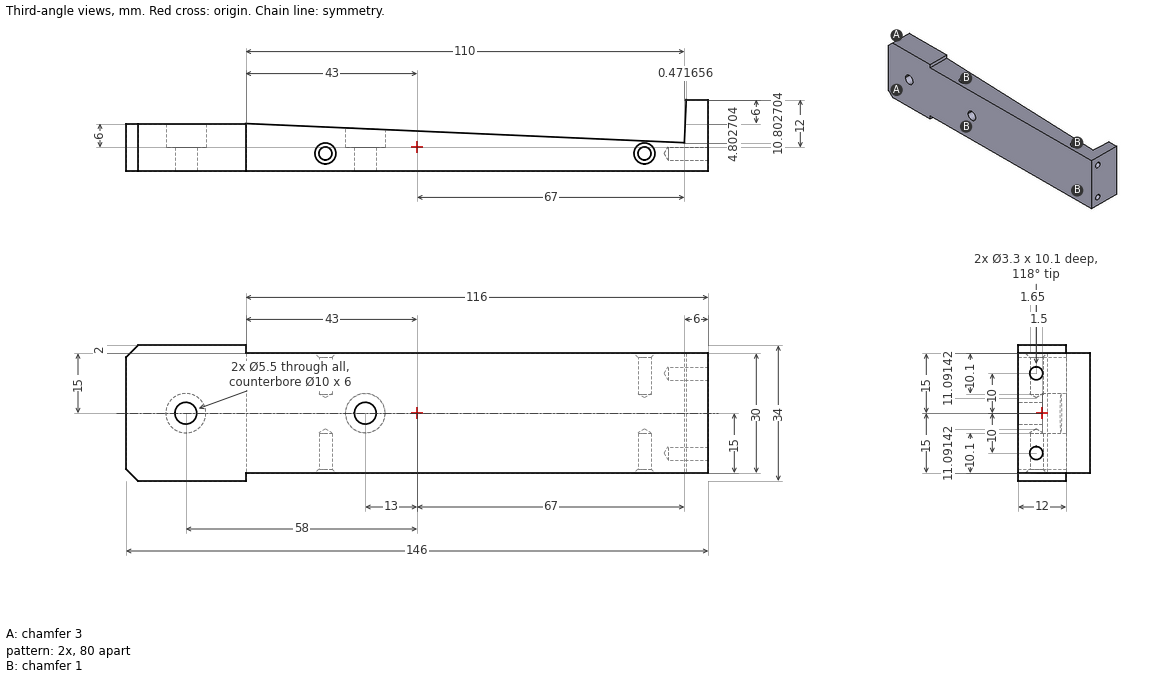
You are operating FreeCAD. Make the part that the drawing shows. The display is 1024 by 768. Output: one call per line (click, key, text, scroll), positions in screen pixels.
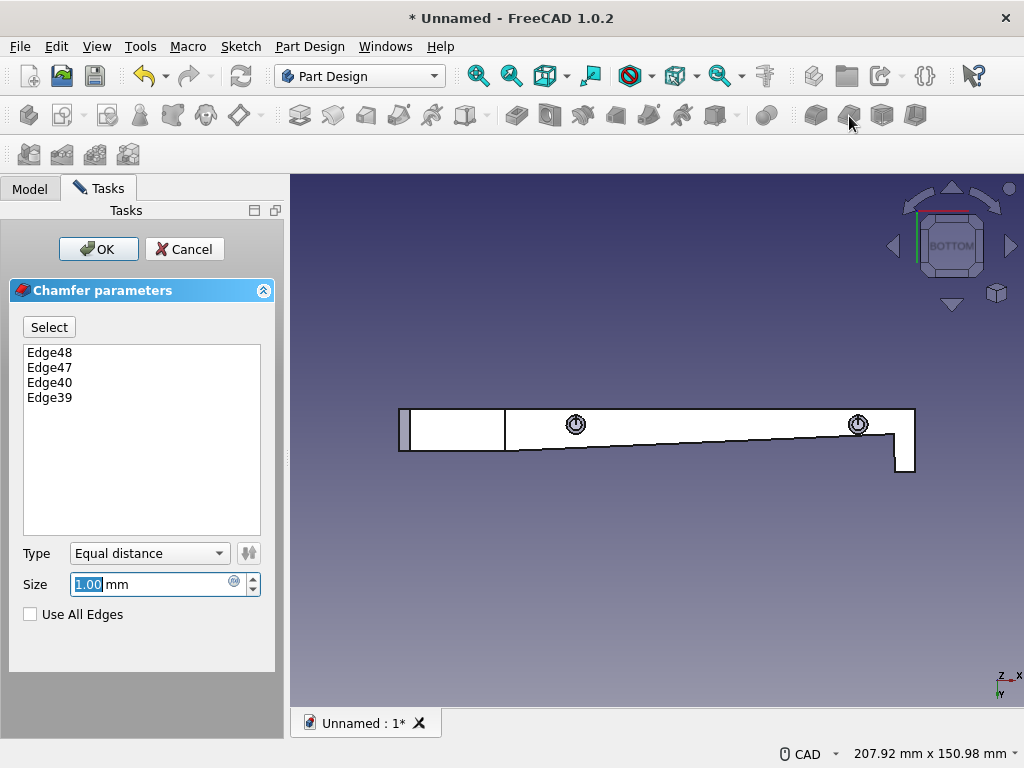
text(1)
key(Tab)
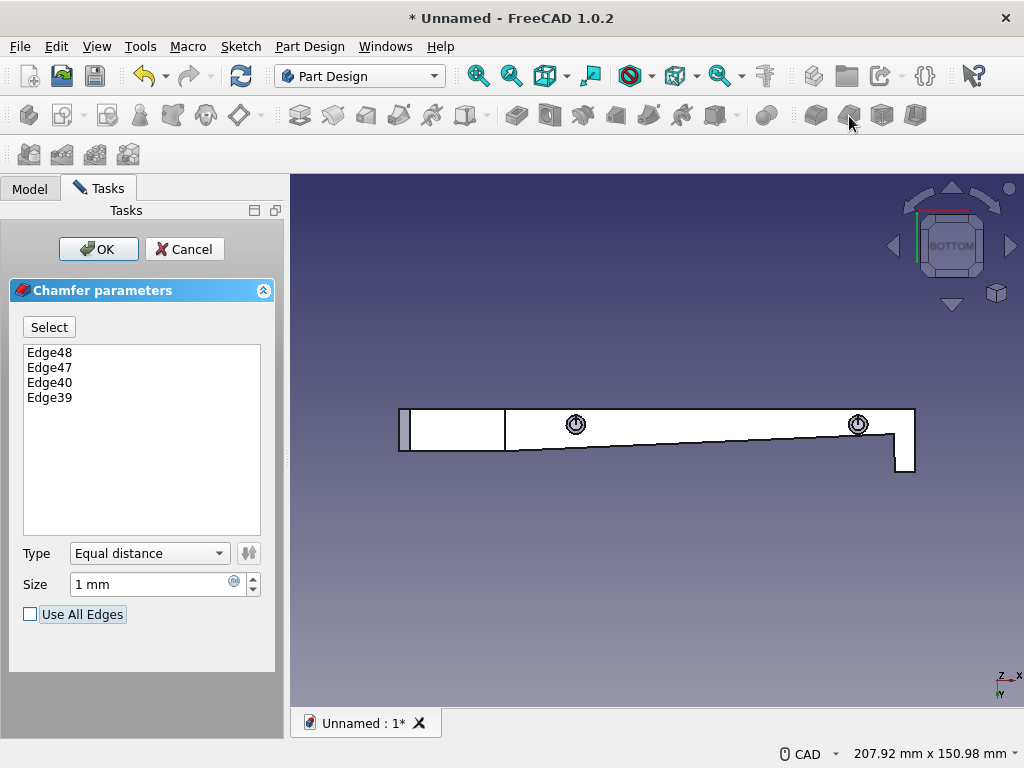
click(99, 249)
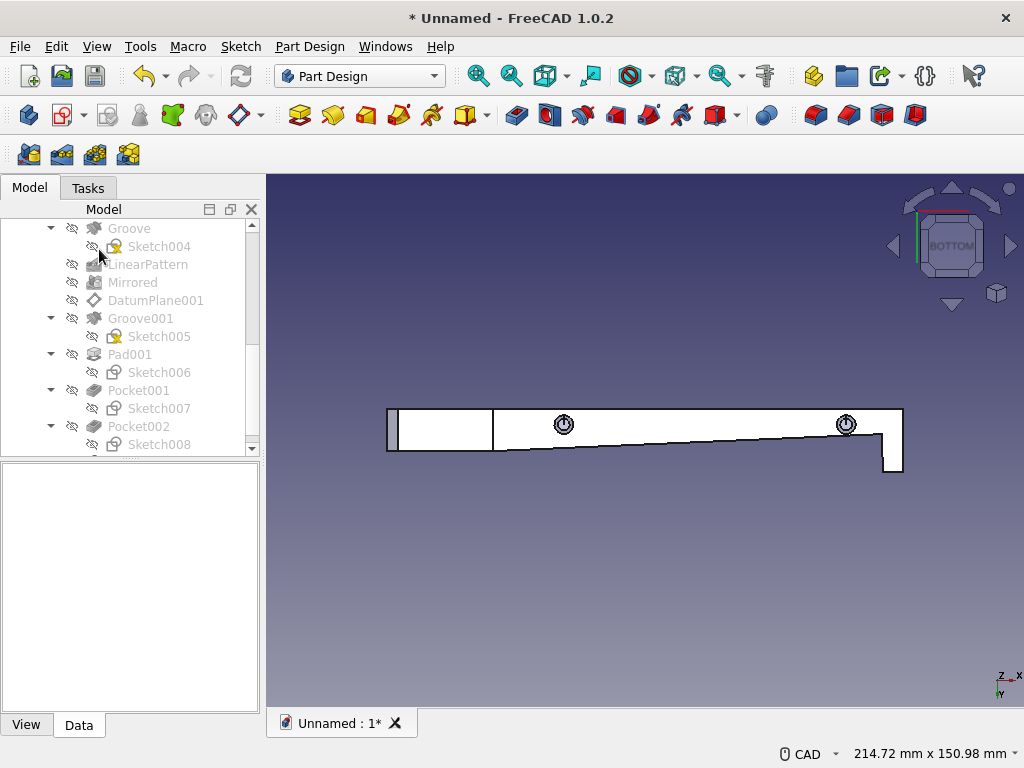
key(0)